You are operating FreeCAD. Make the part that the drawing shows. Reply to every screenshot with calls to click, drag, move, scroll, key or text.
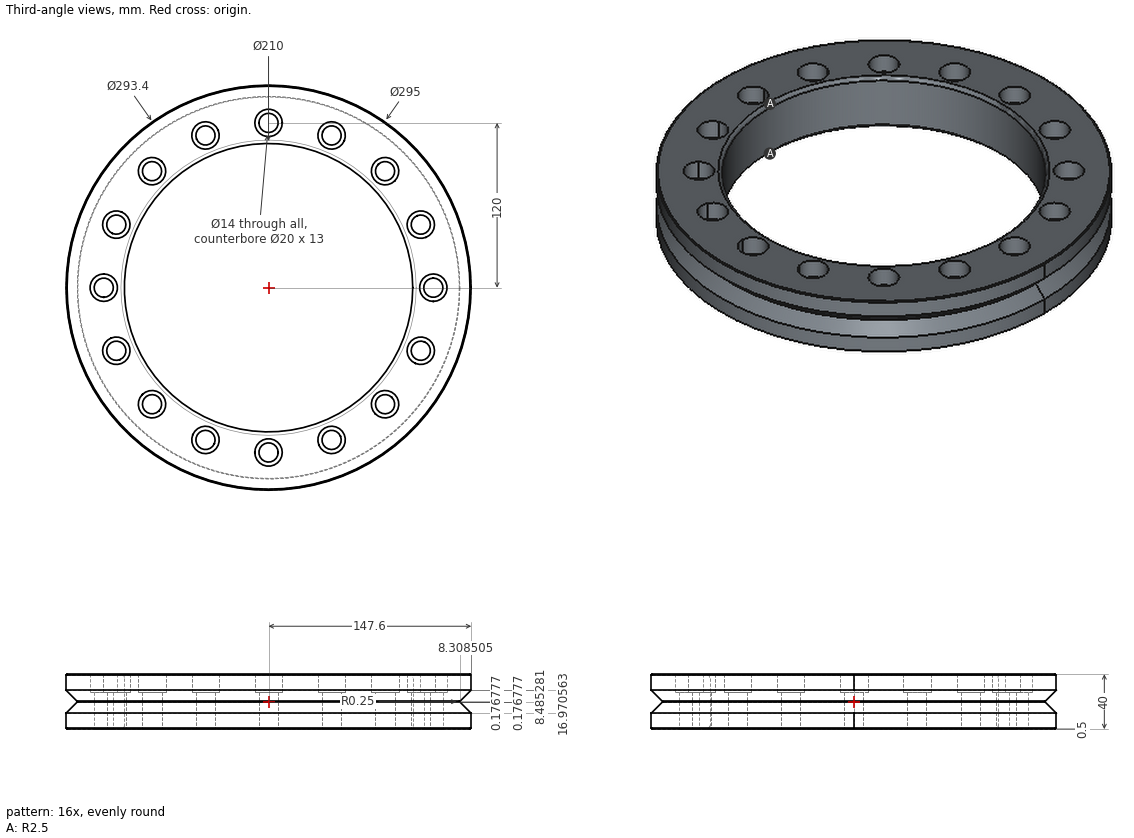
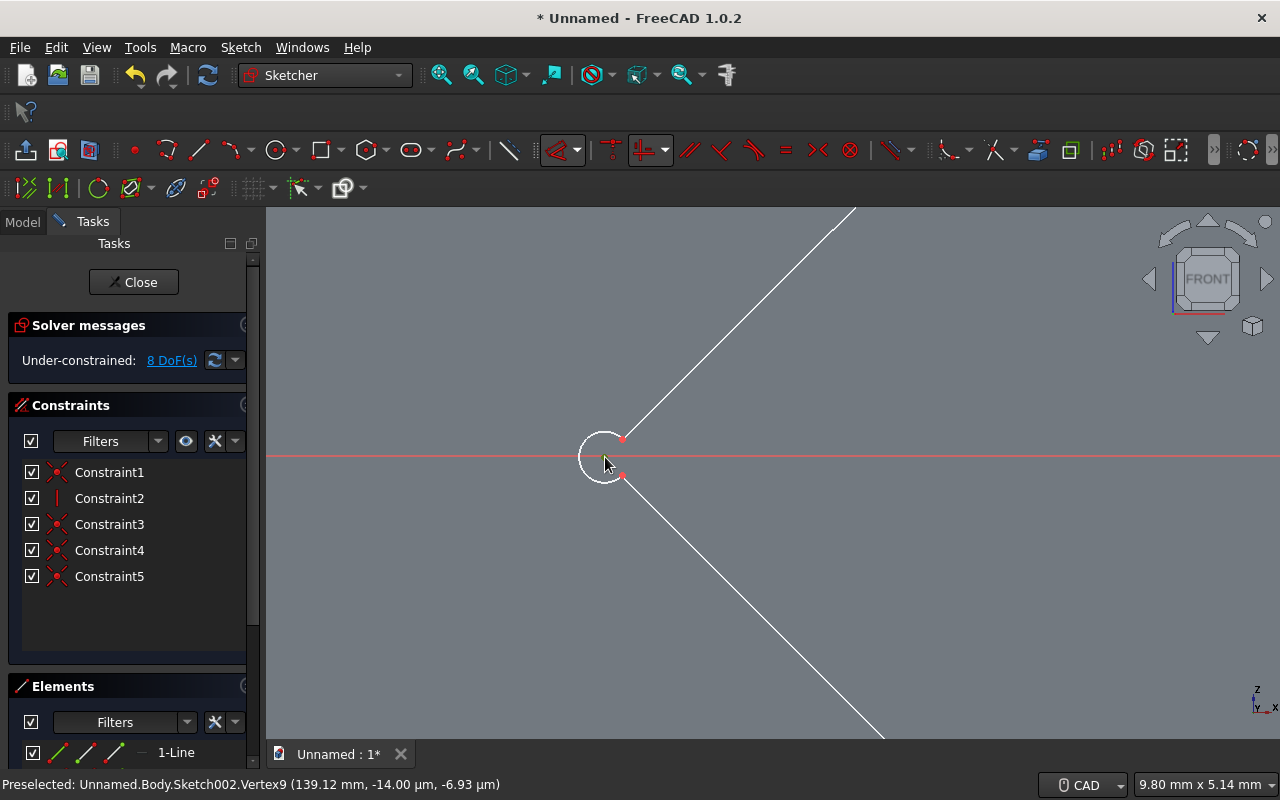
click(353, 456)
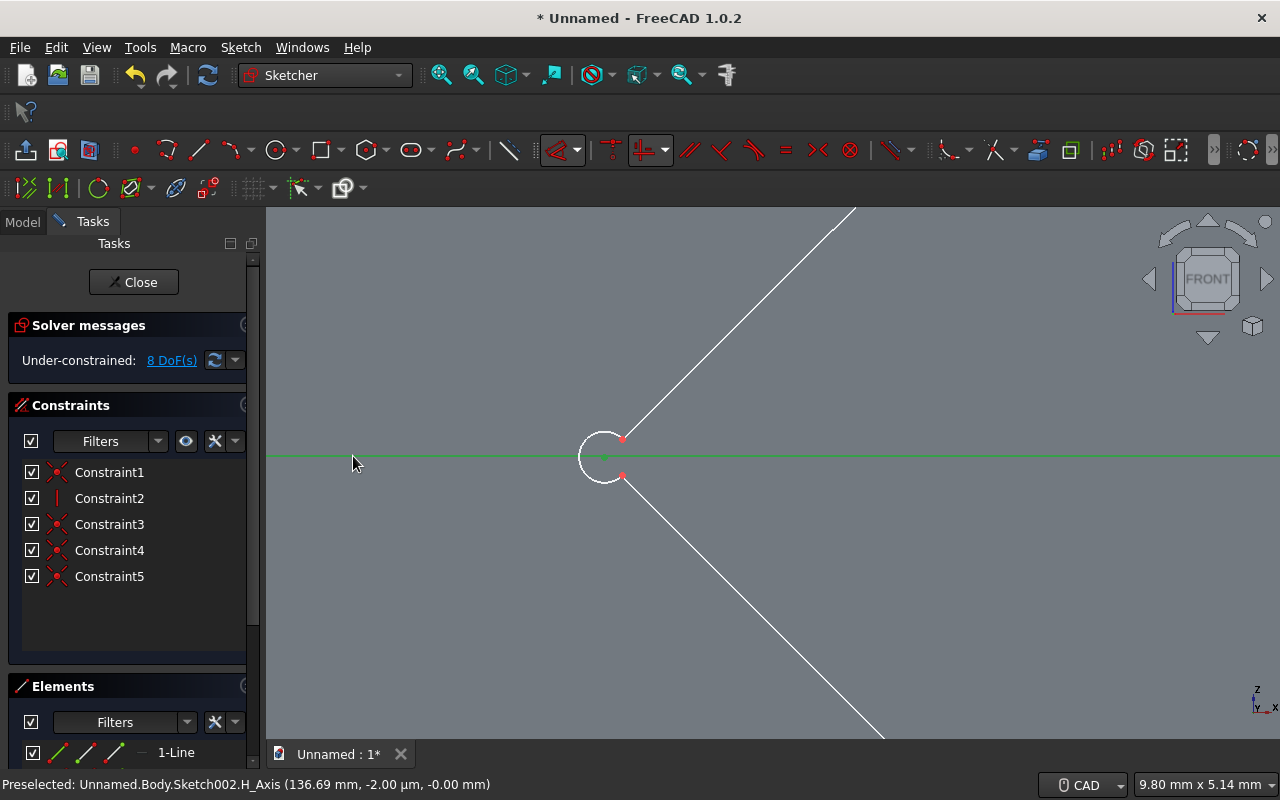
click(612, 150)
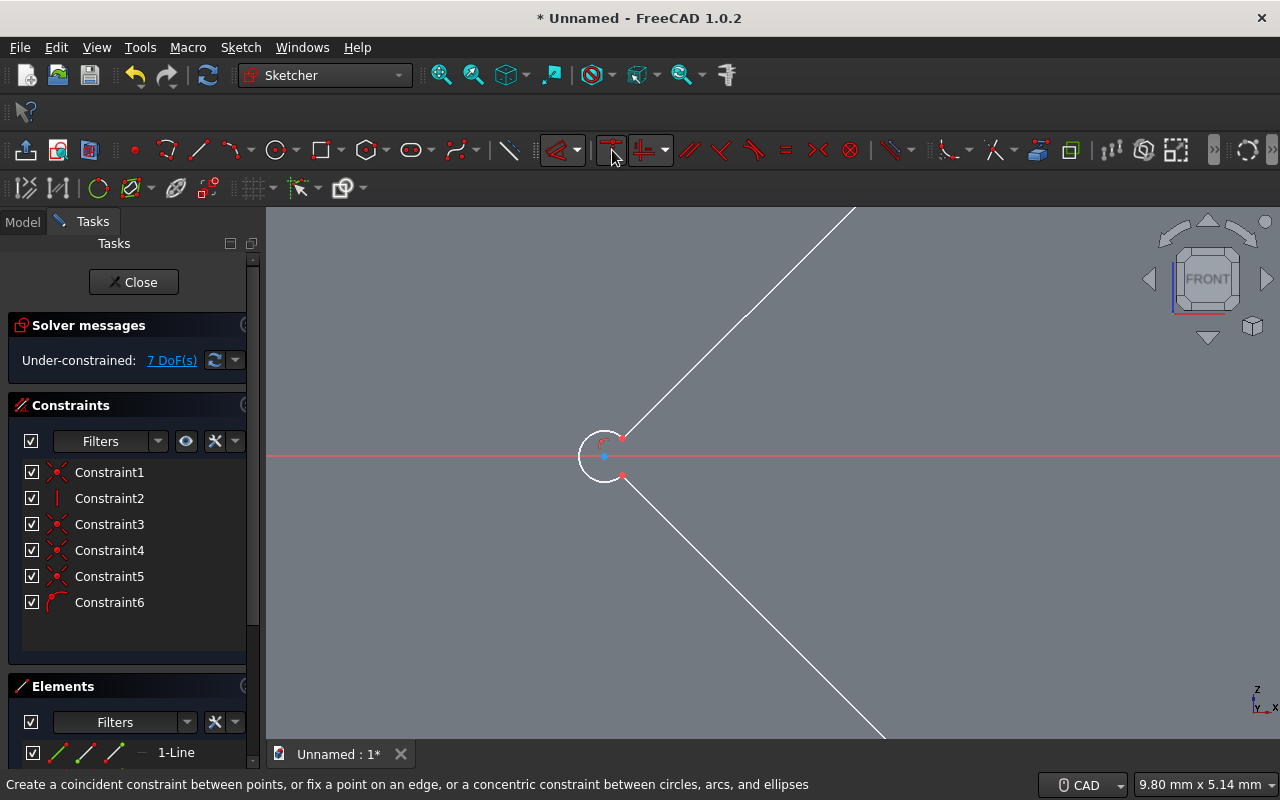
click(556, 150)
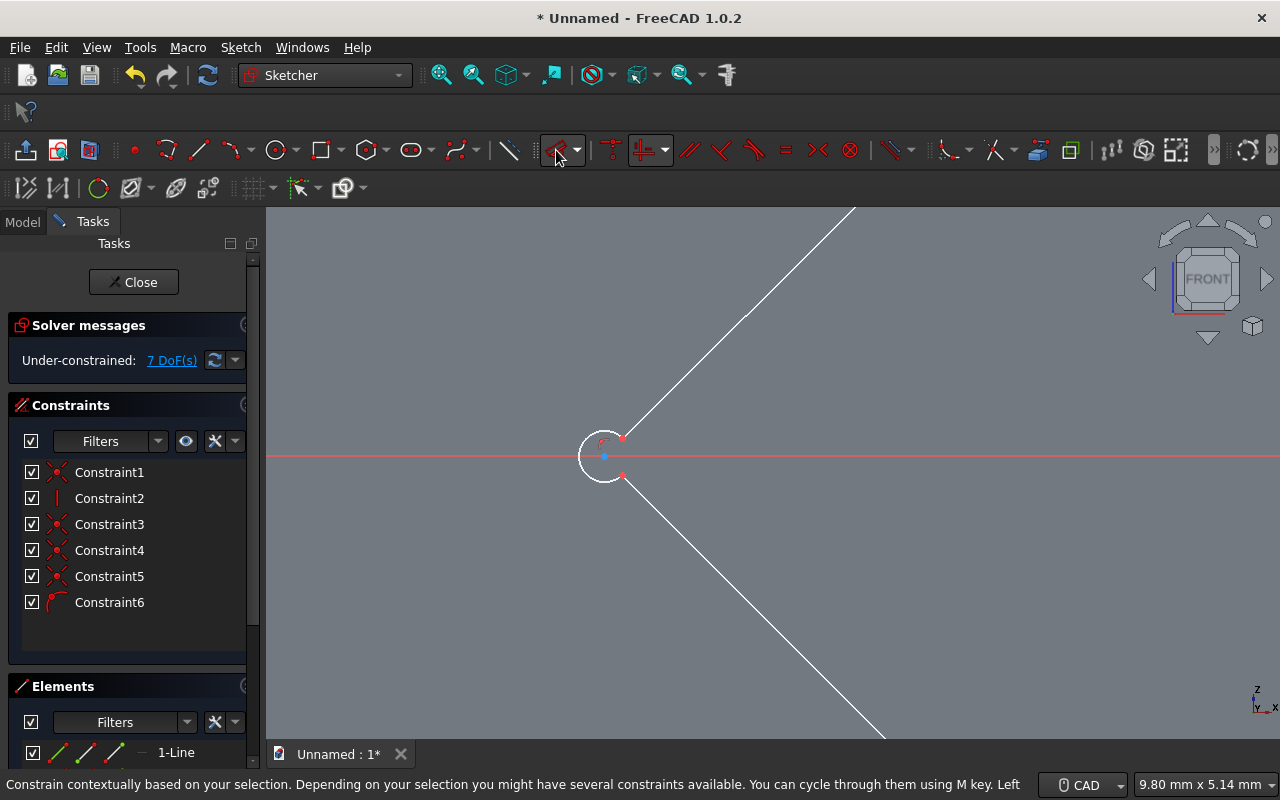
scroll(590, 436, up, 3)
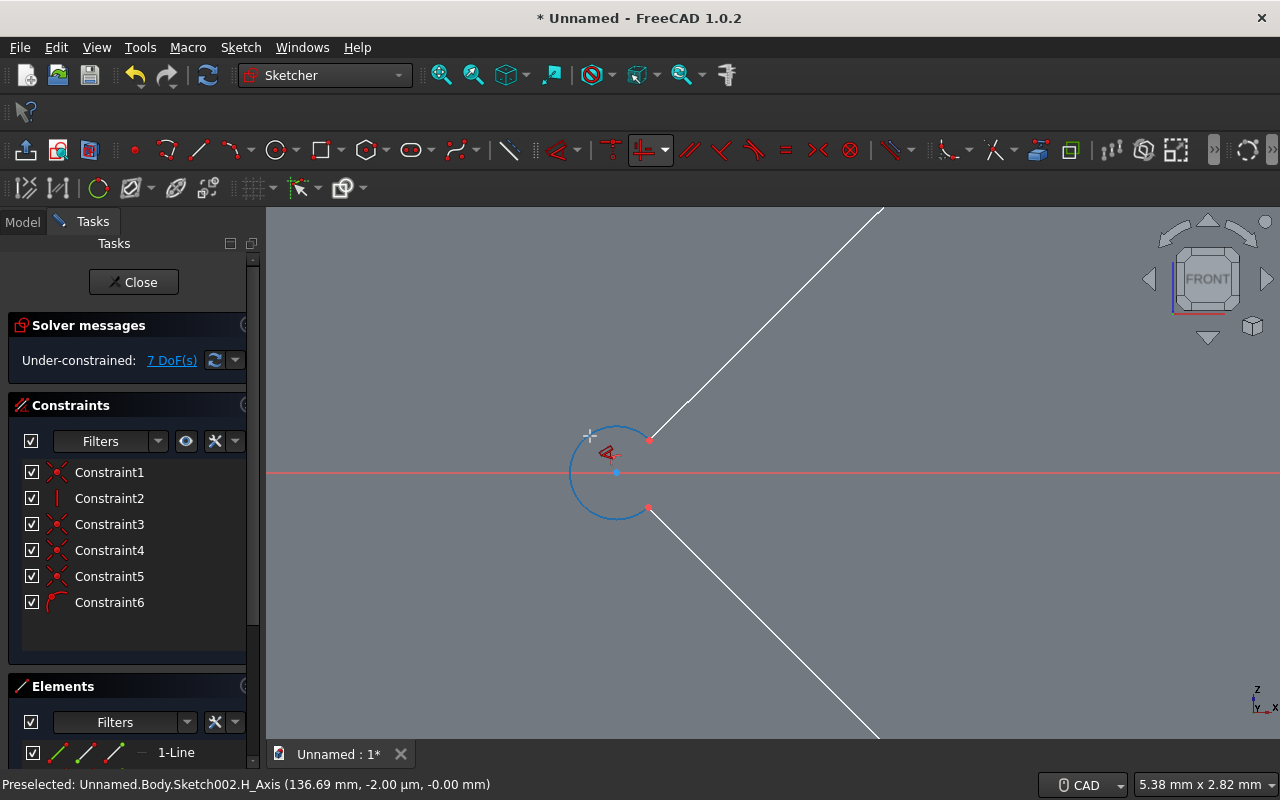
click(590, 435)
click(572, 409)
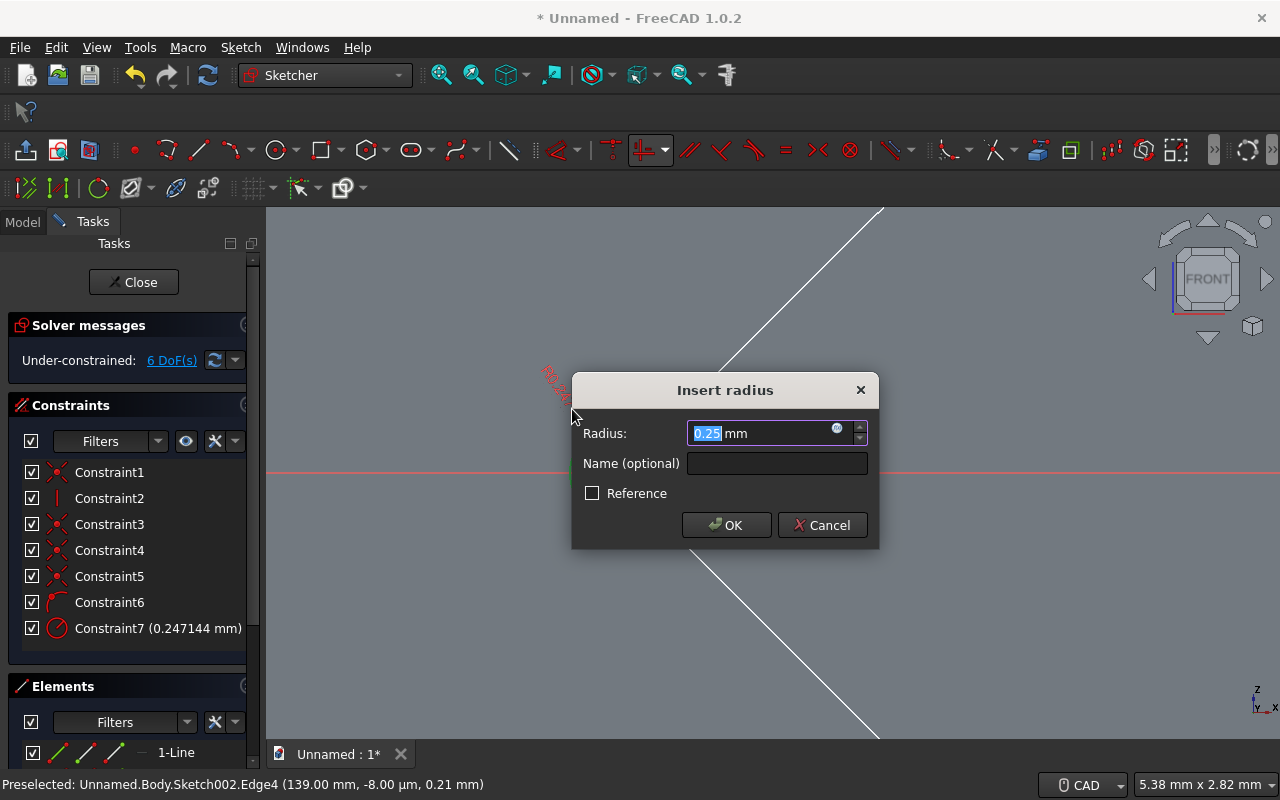
text(0.25)
key(Return)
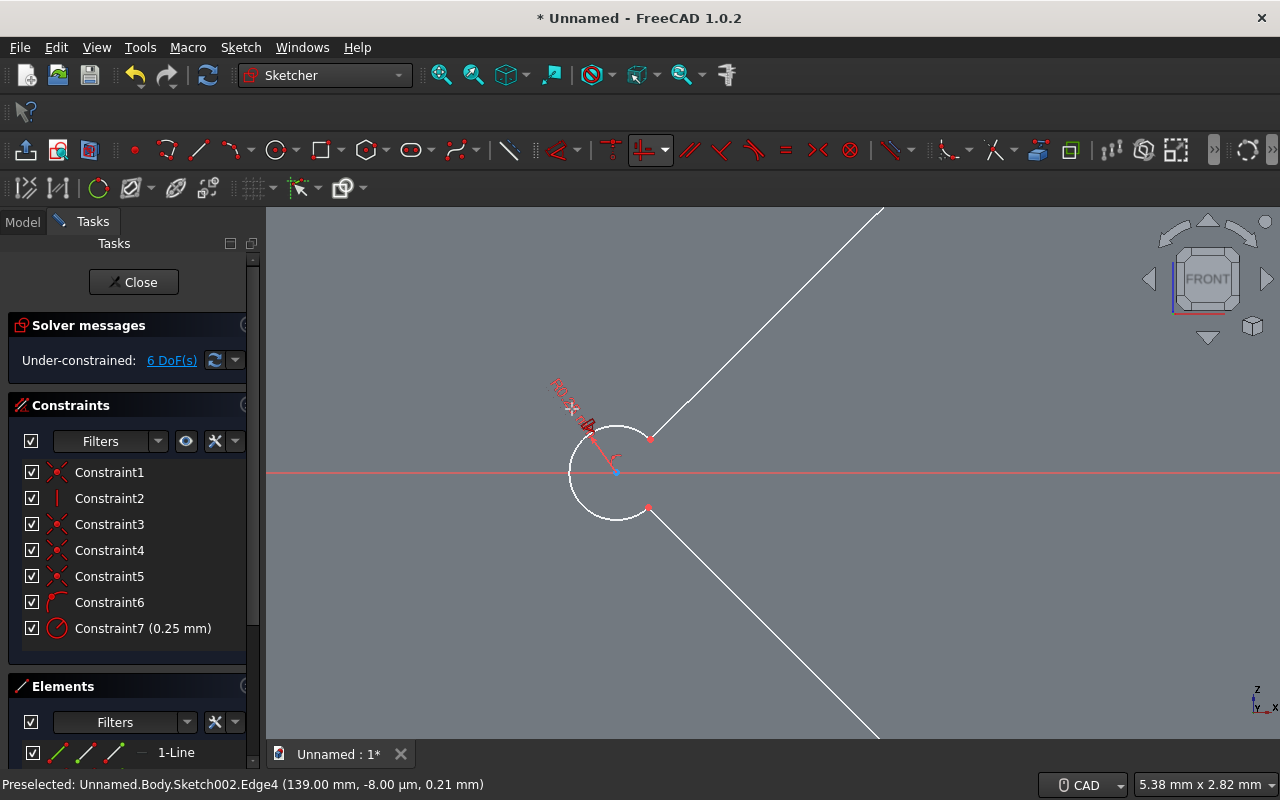
scroll(619, 473, down, 11)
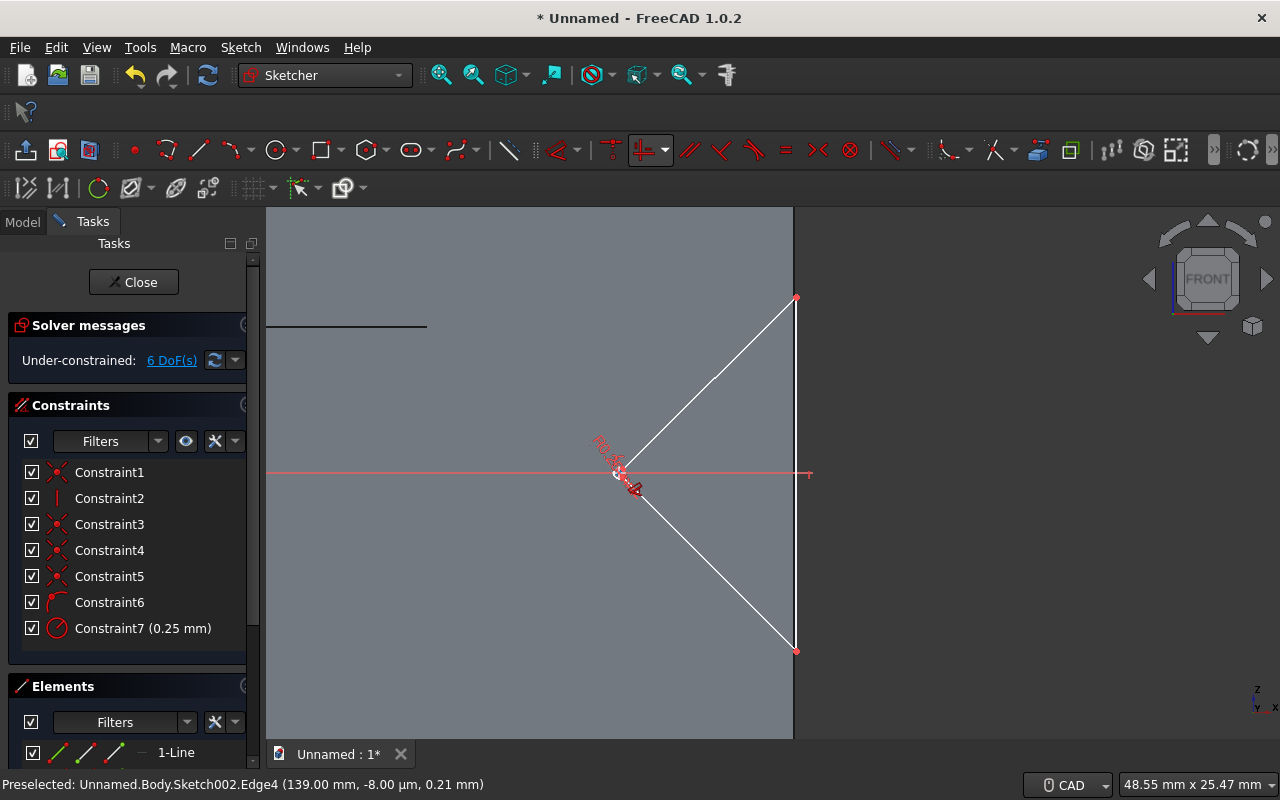
click(796, 297)
click(545, 263)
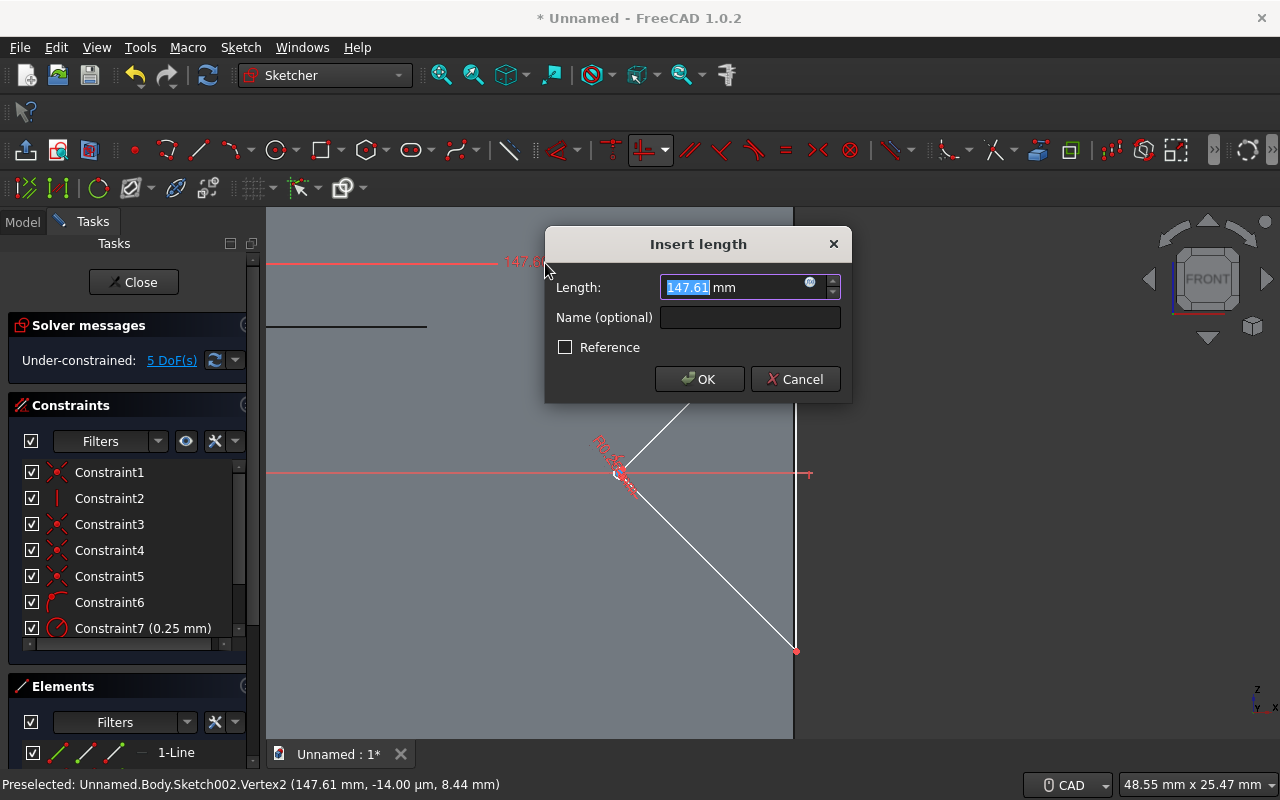
text(147.6)
key(Return)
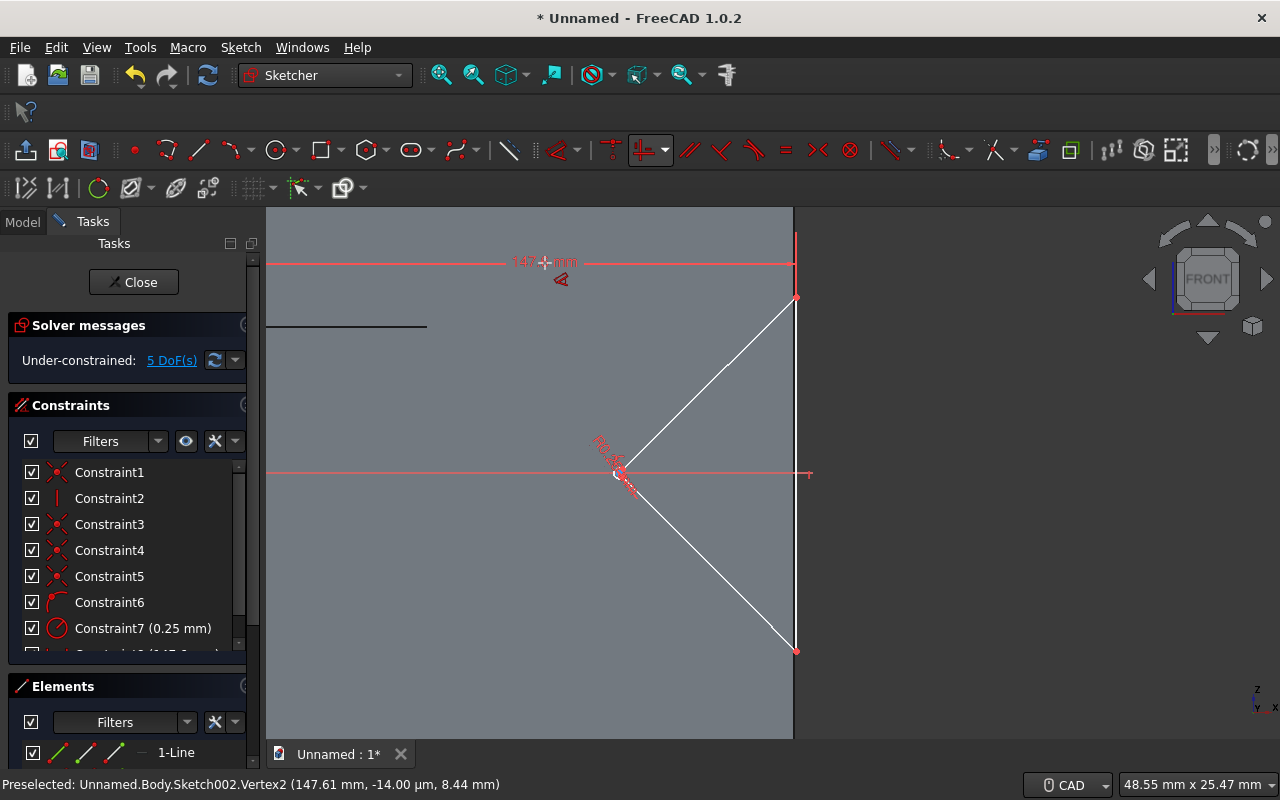
click(796, 403)
click(830, 393)